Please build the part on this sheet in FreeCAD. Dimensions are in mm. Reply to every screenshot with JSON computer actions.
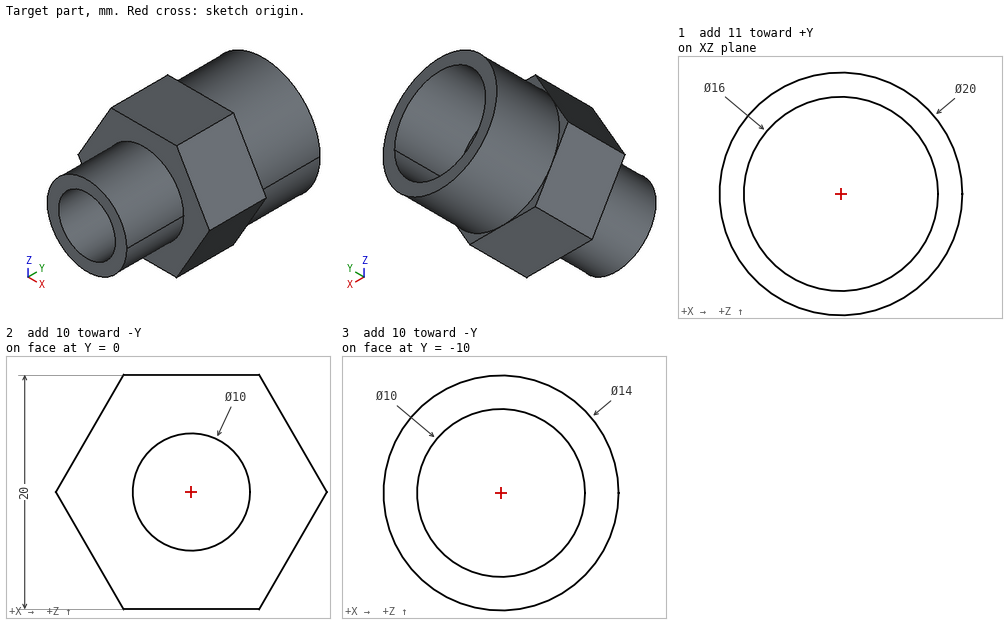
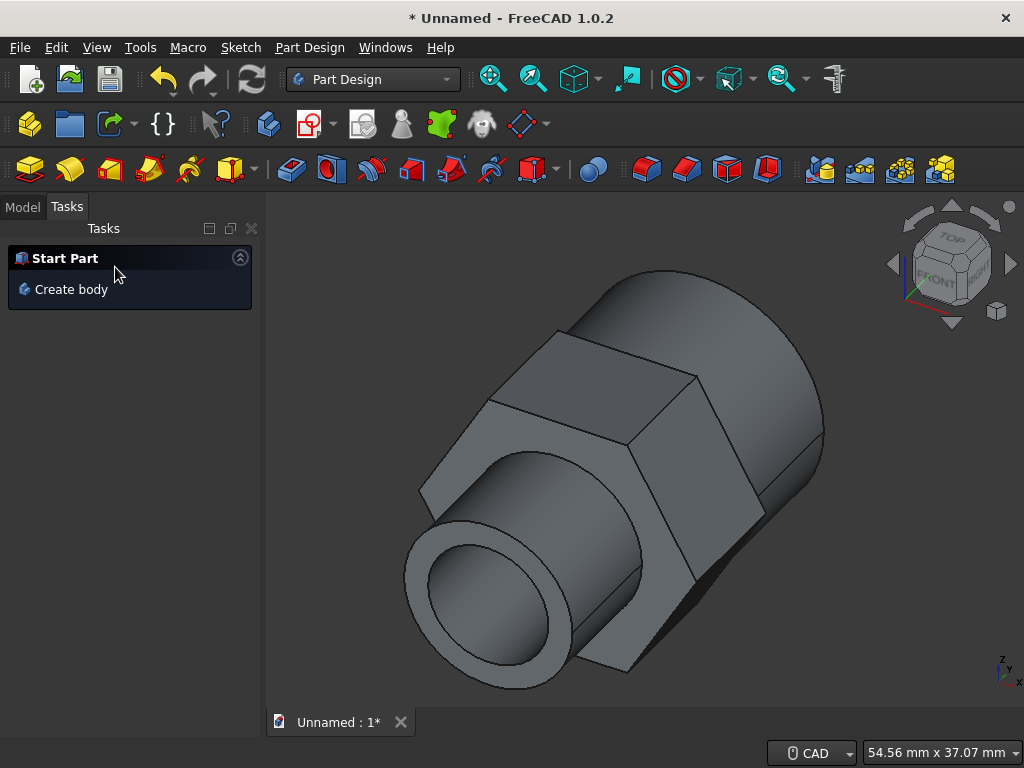
{"action": "key", "text": "0"}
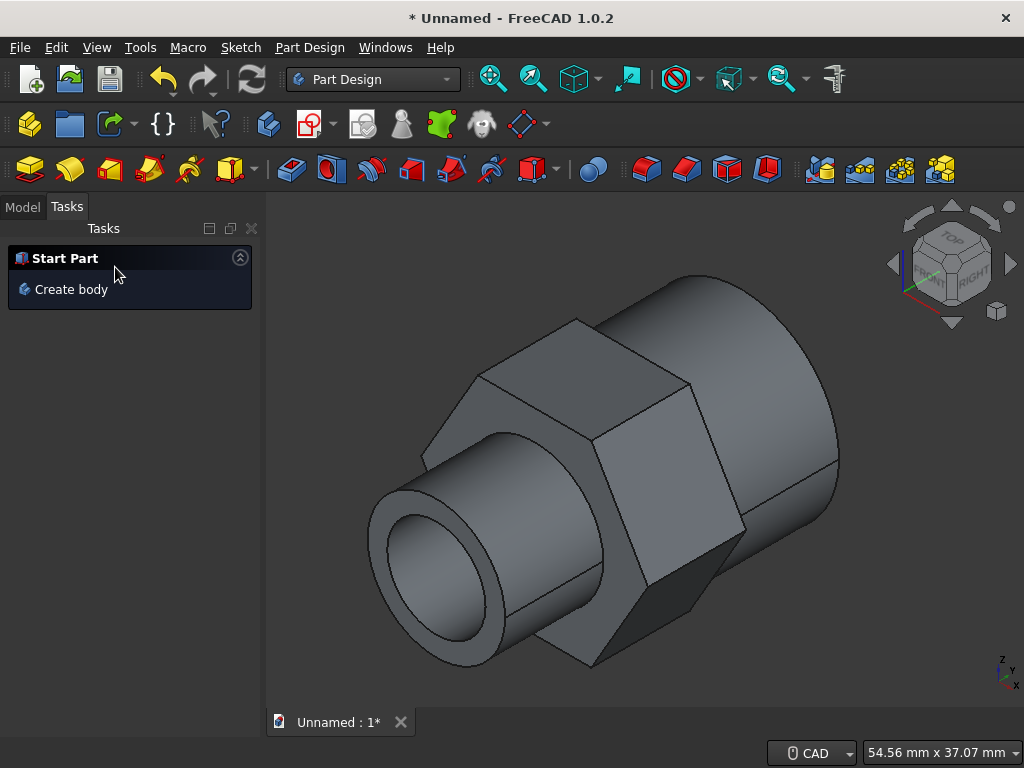
{"action": "left_click", "coordinate": [494, 80]}